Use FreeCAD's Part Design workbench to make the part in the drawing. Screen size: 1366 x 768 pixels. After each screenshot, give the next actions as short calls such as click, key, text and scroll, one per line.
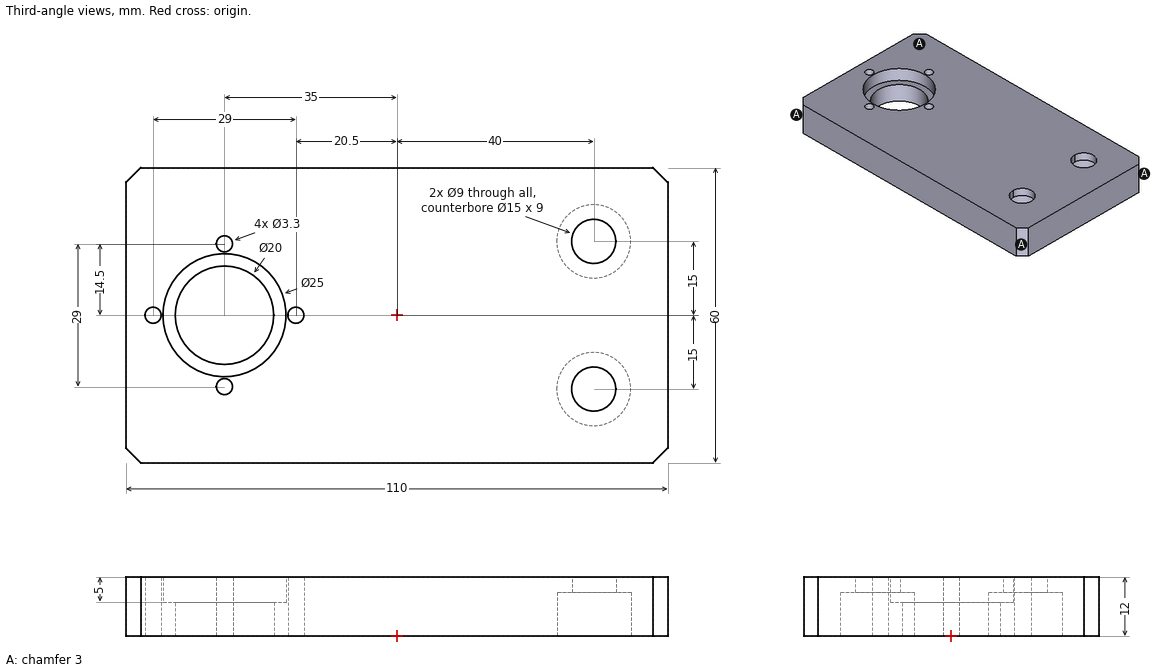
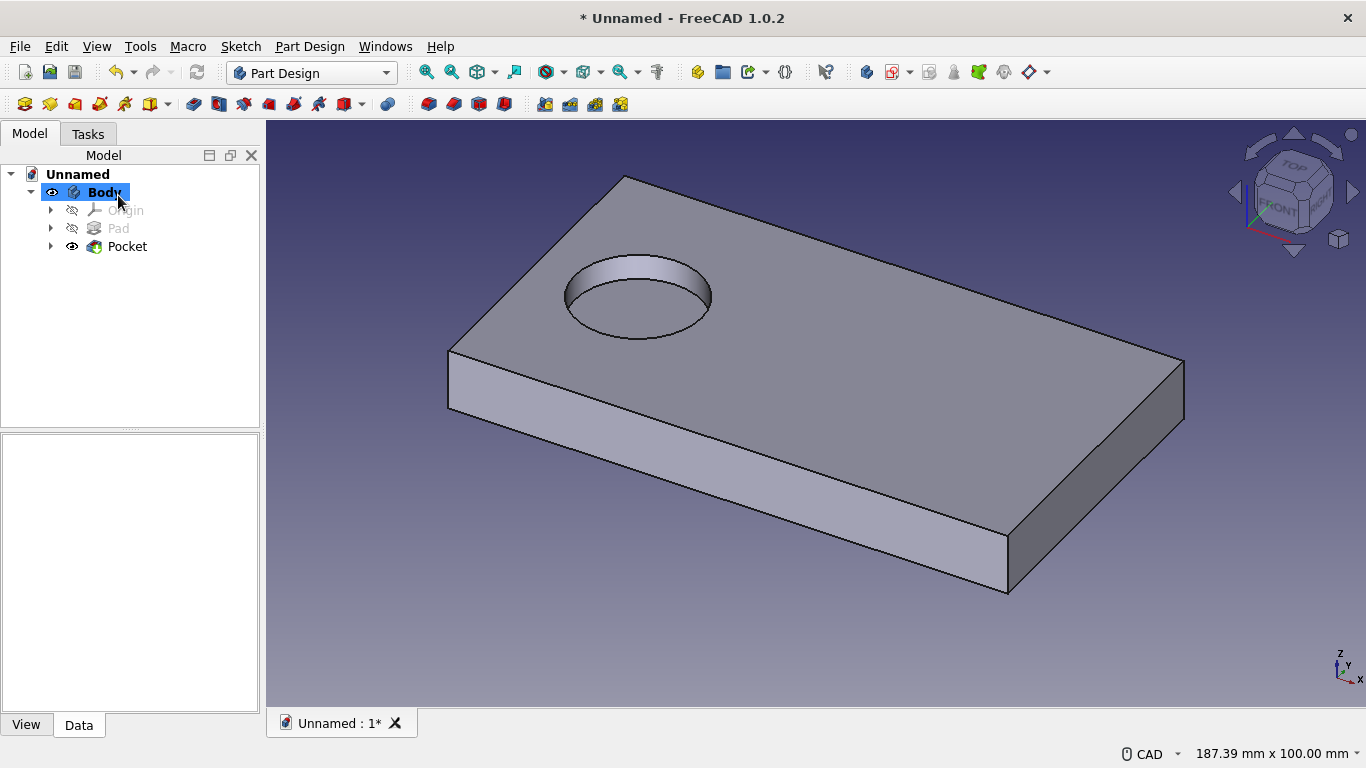
click(896, 381)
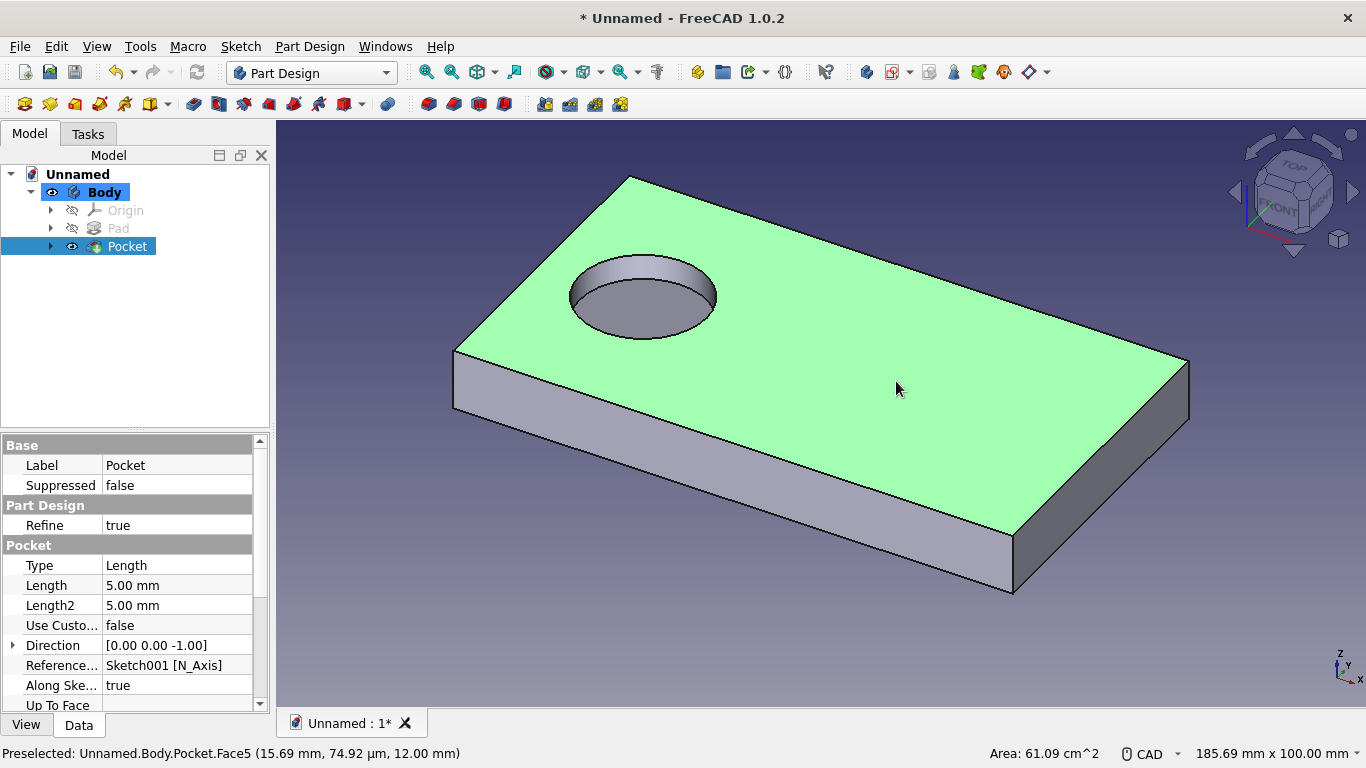
click(892, 72)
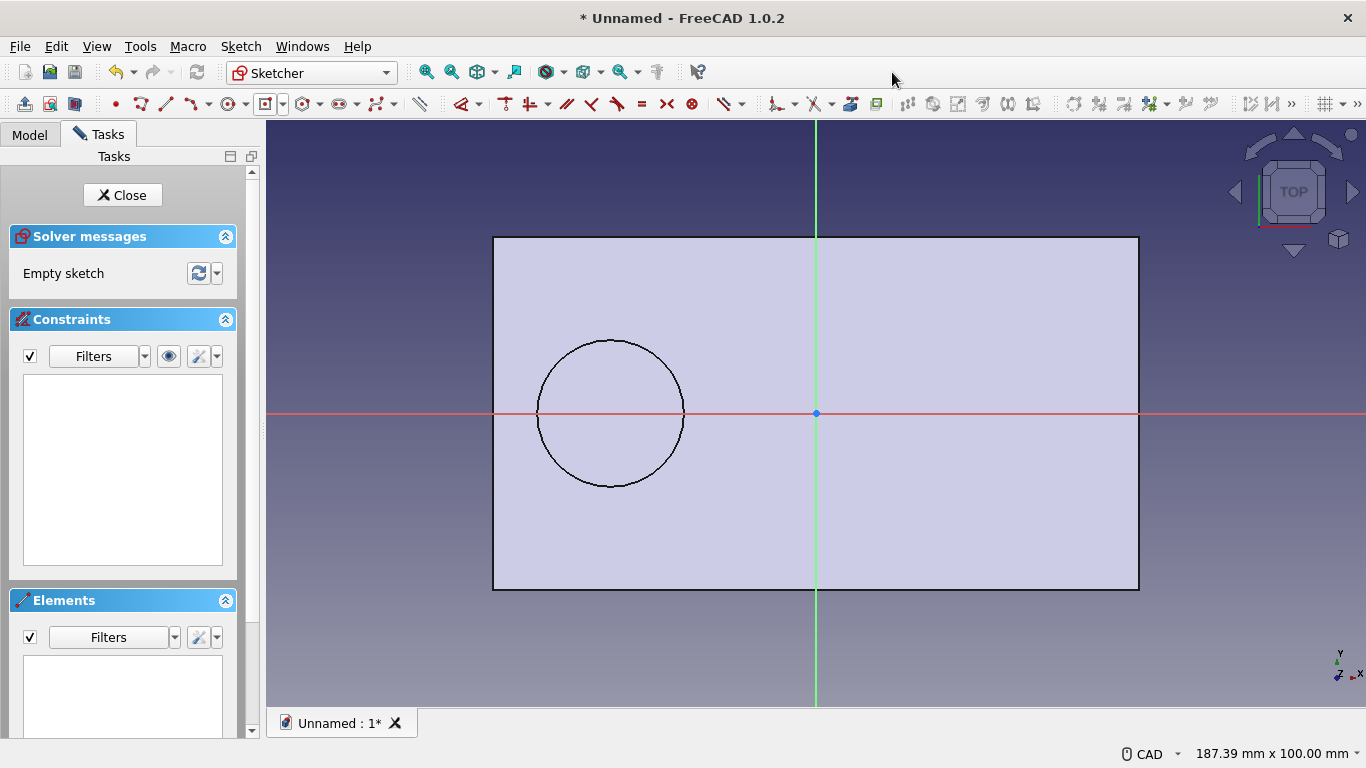
scroll(632, 413, up, 4)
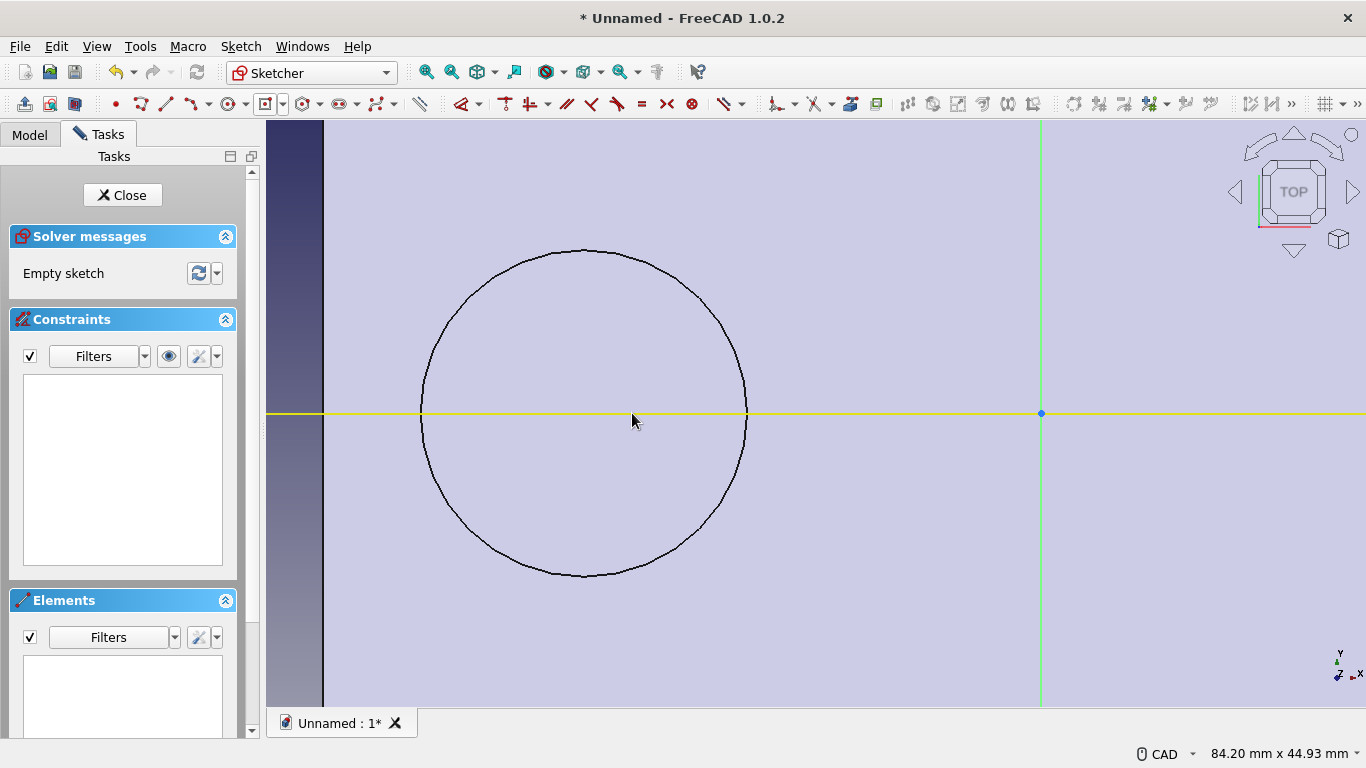
click(228, 104)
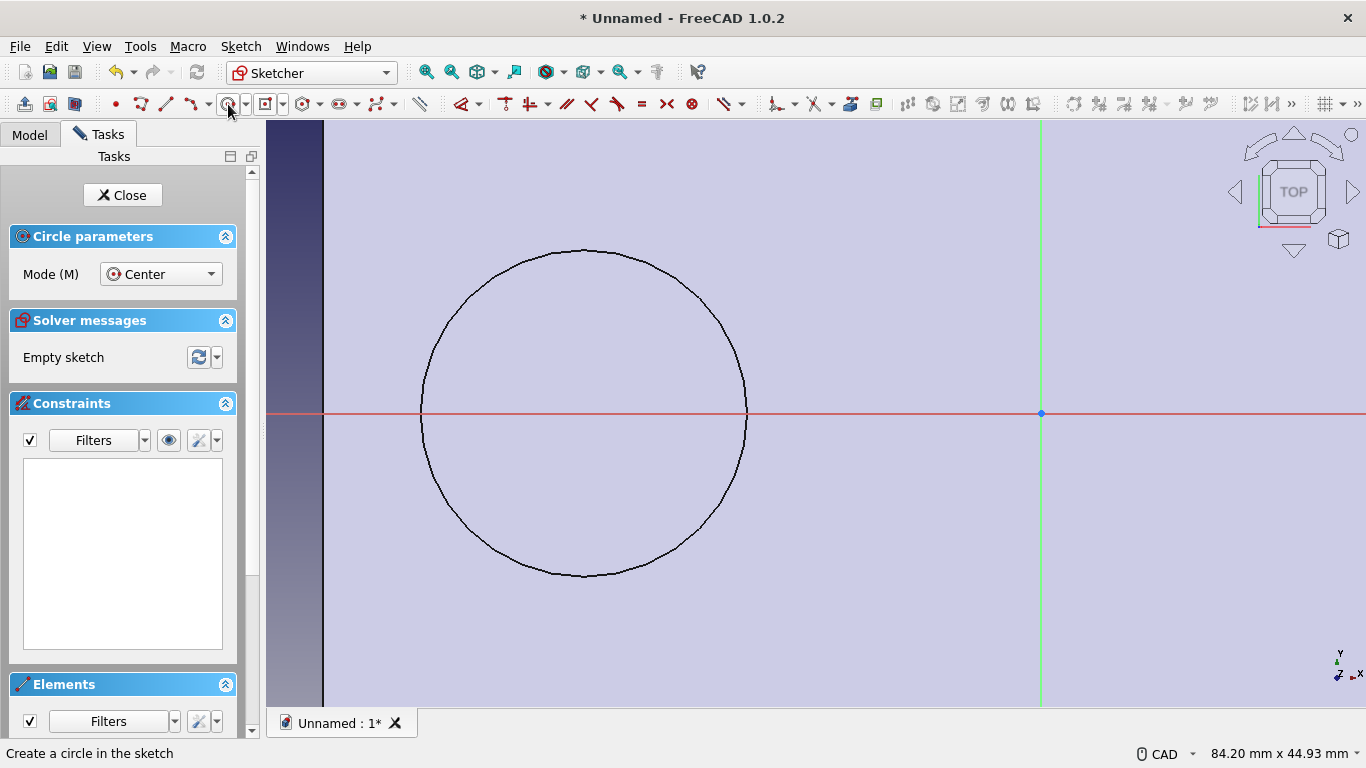
click(584, 414)
click(676, 321)
key(Escape)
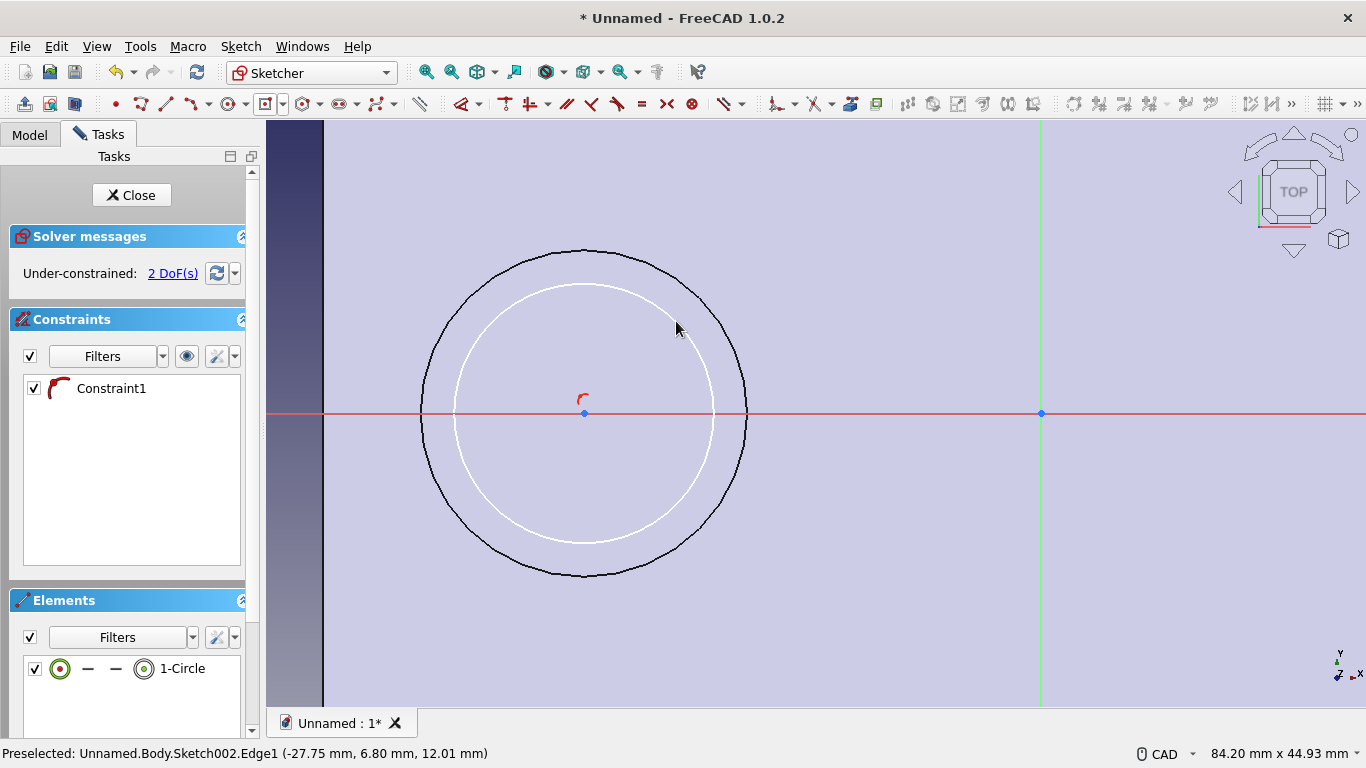
click(460, 104)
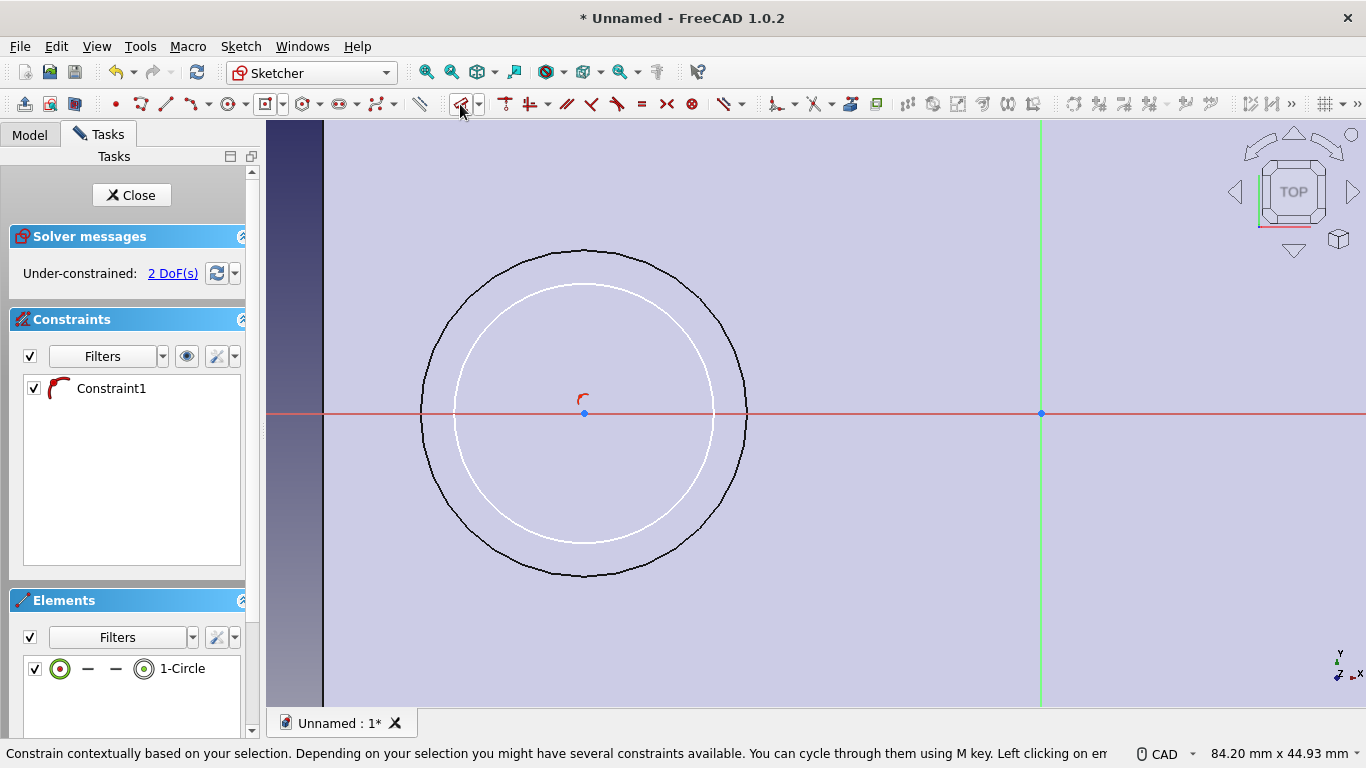
click(675, 321)
click(697, 298)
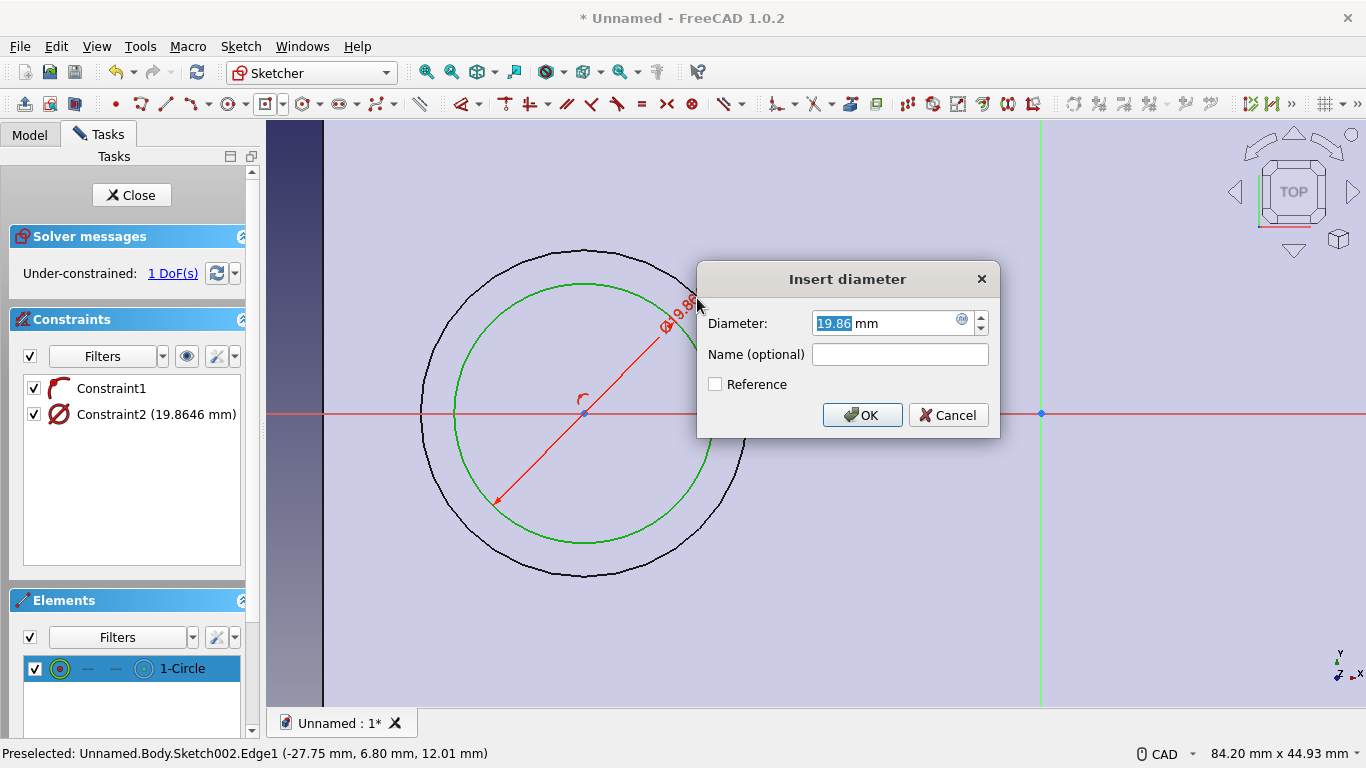
text(20)
key(Return)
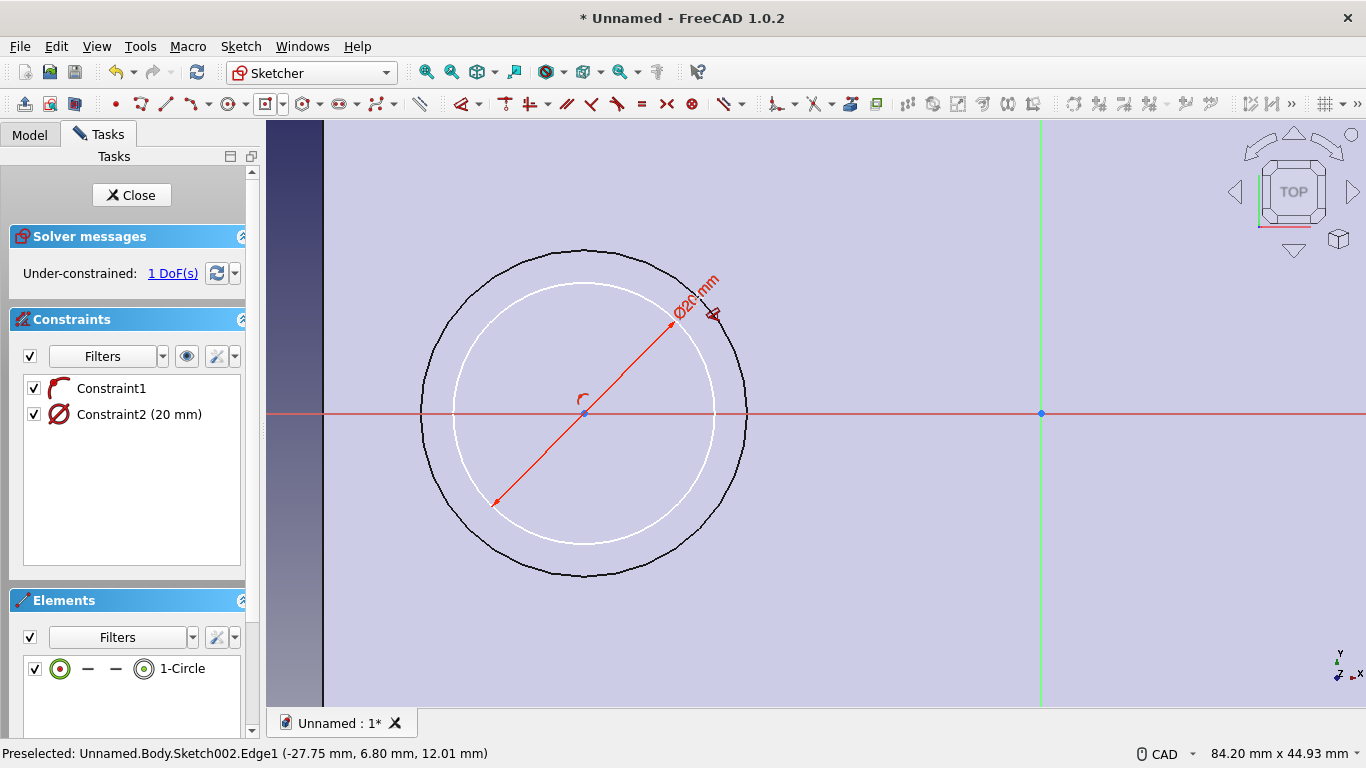
click(584, 414)
click(813, 448)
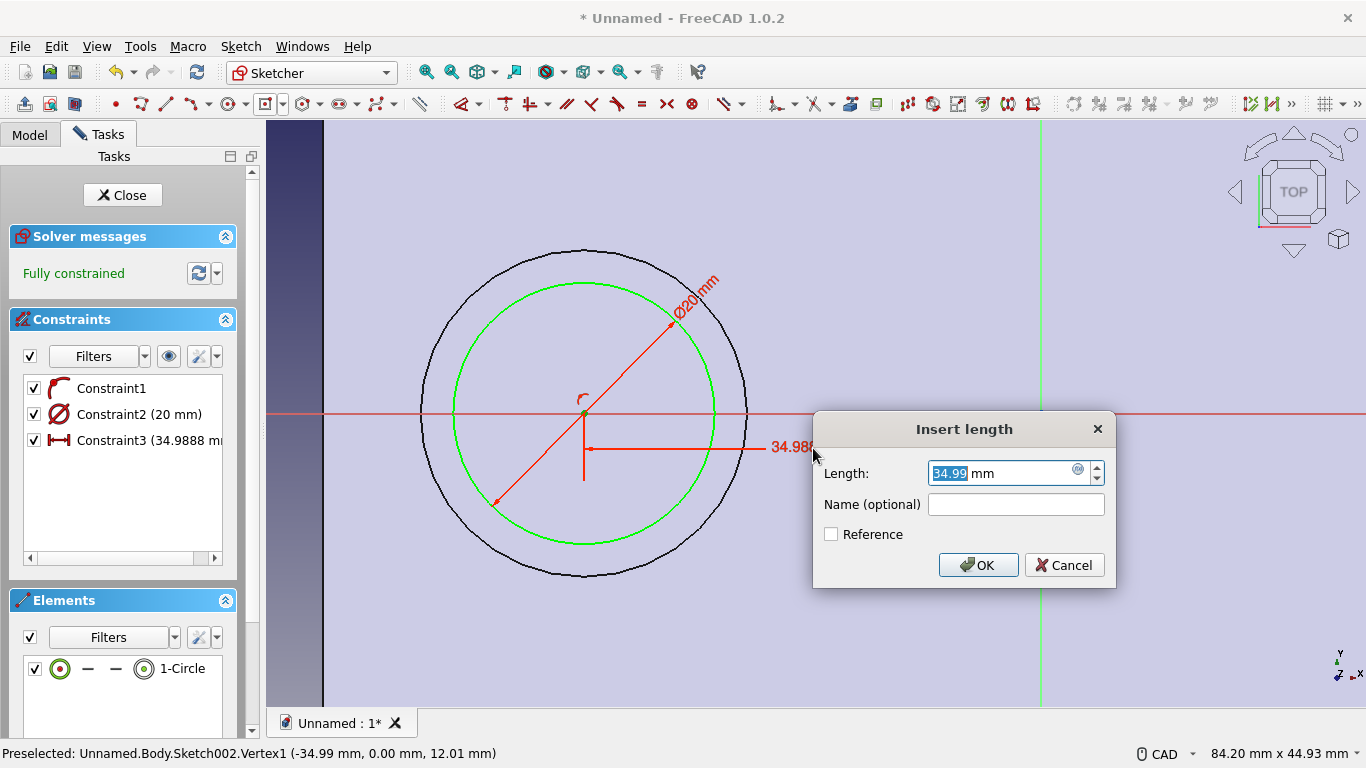
text(35)
key(Return)
key(Escape)